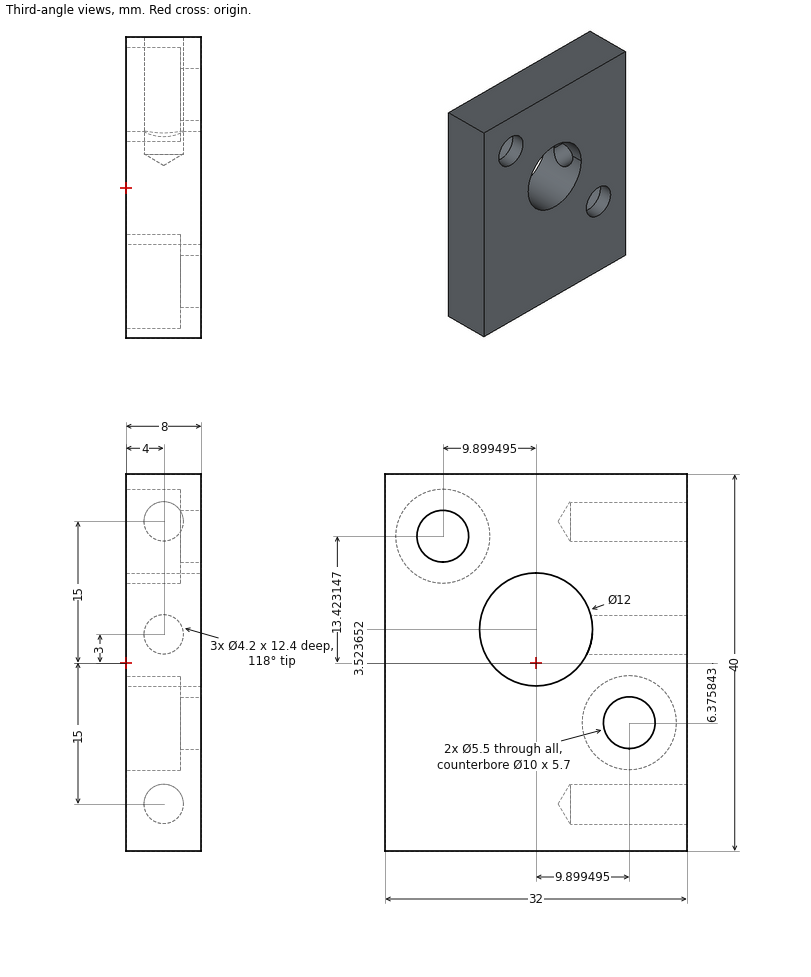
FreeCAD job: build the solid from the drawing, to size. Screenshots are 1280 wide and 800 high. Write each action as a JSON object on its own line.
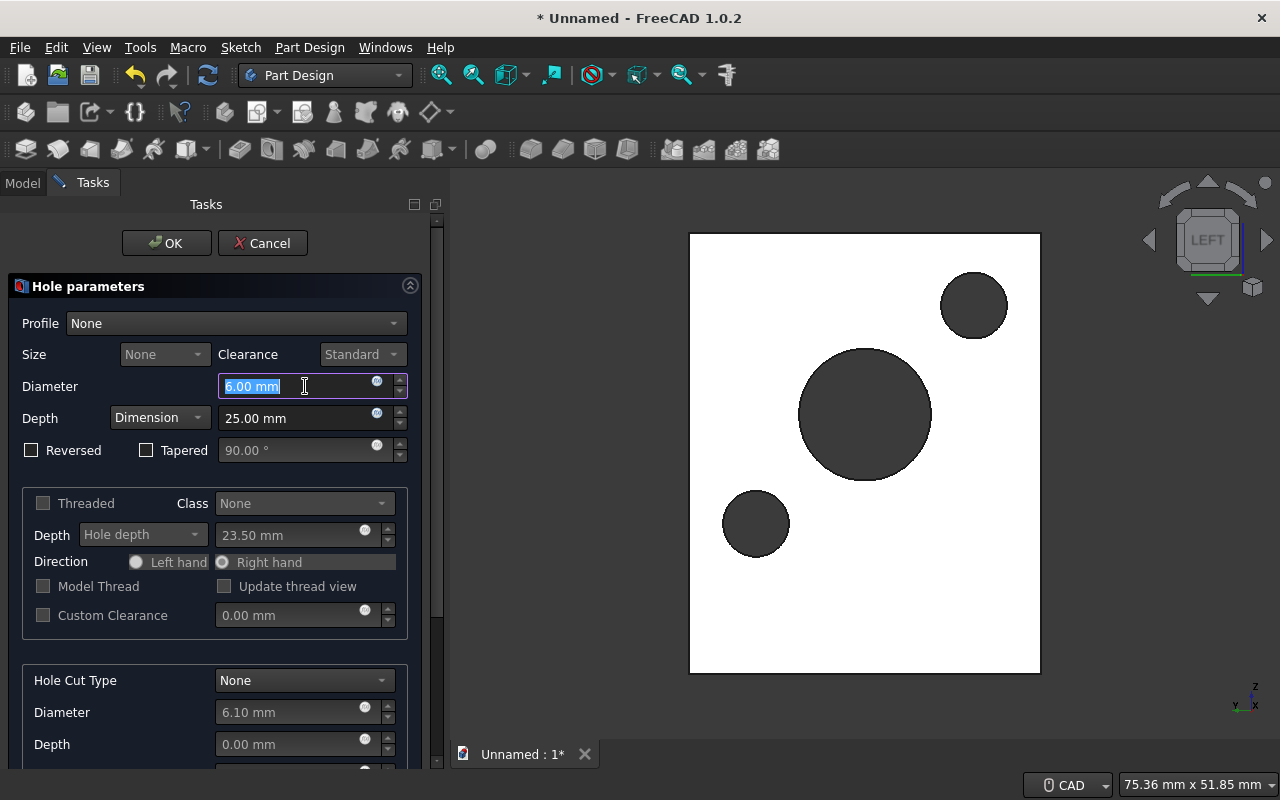
{"action": "type", "text": "5.5"}
{"action": "key", "text": "Tab"}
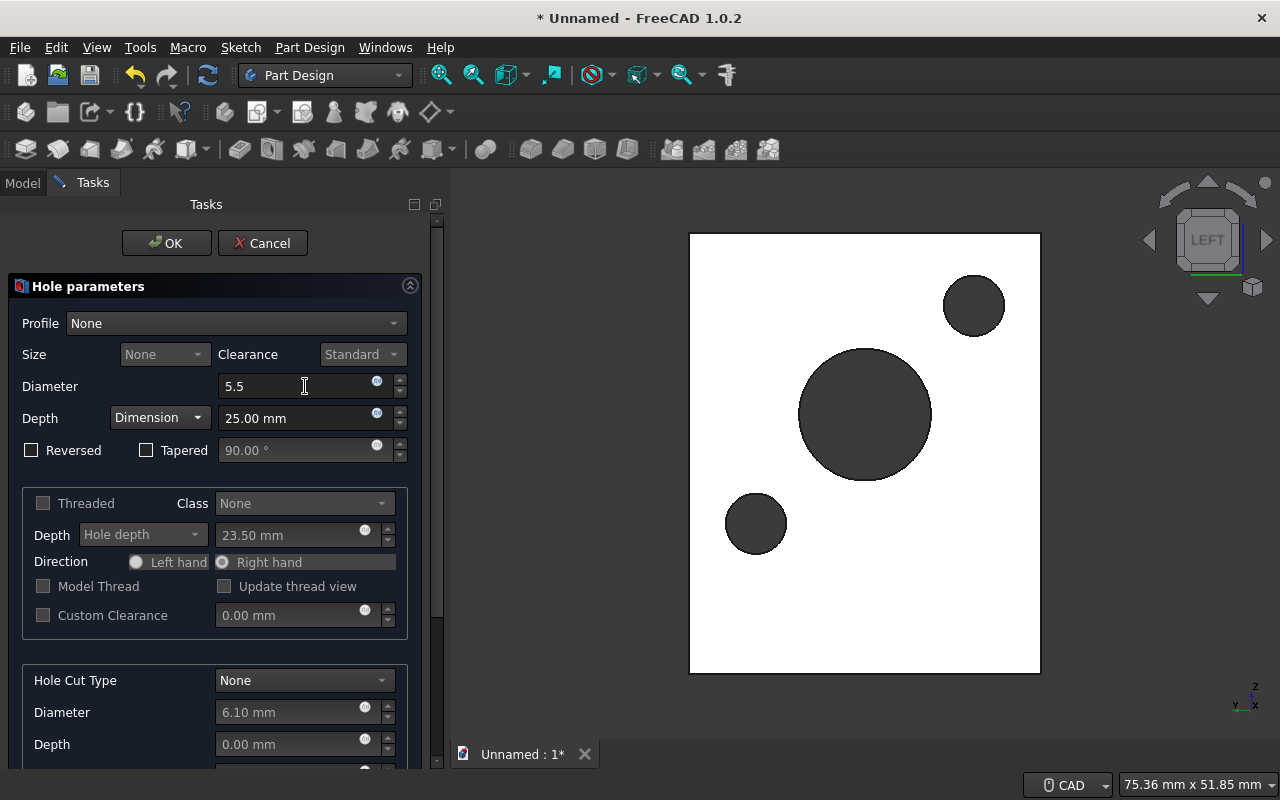
{"action": "left_click", "coordinate": [161, 418]}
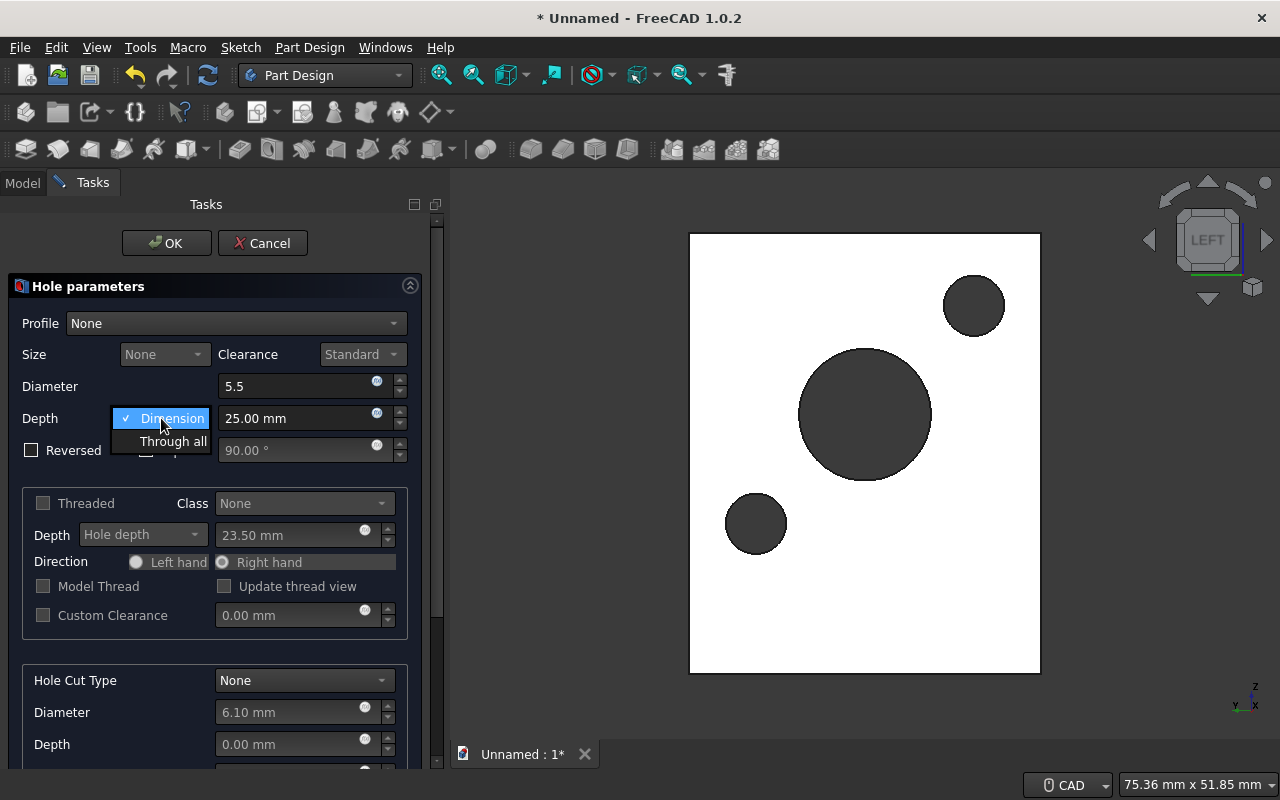
{"action": "left_click", "coordinate": [160, 442]}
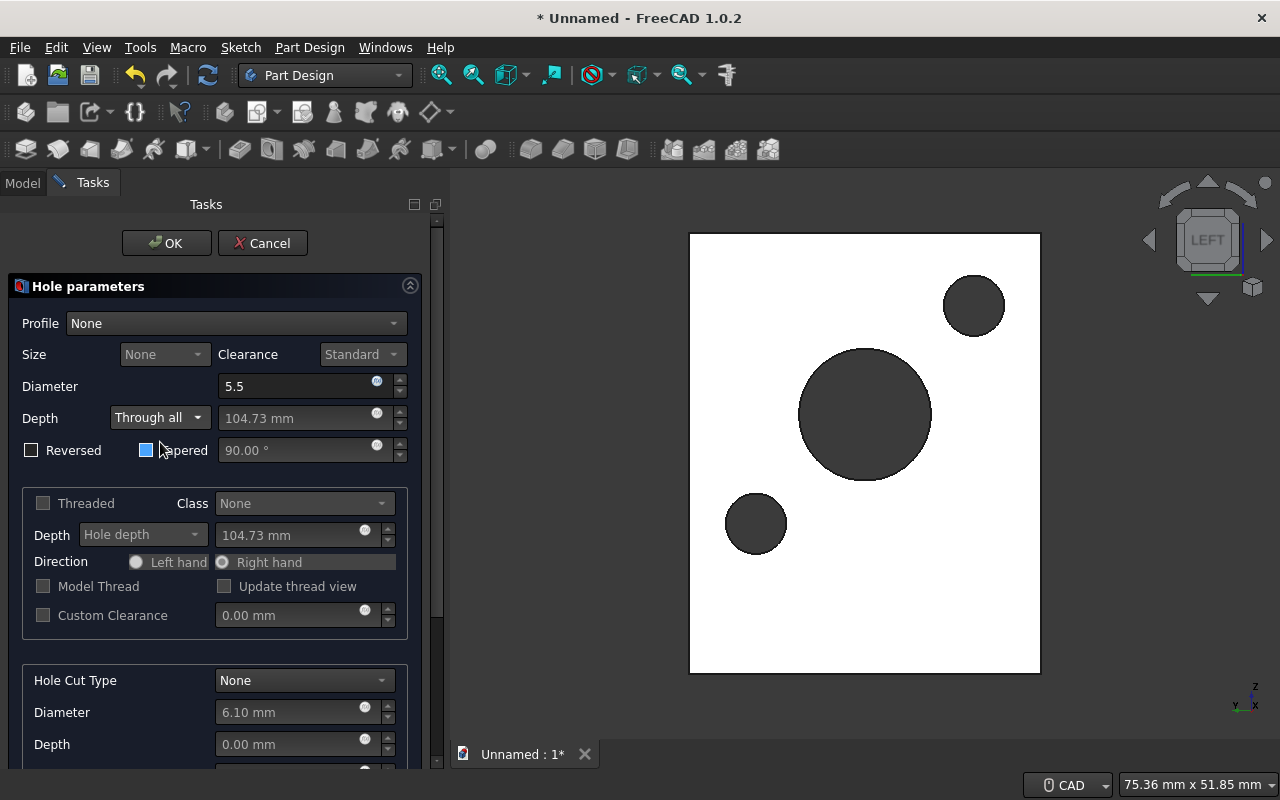
{"action": "left_click", "coordinate": [306, 680]}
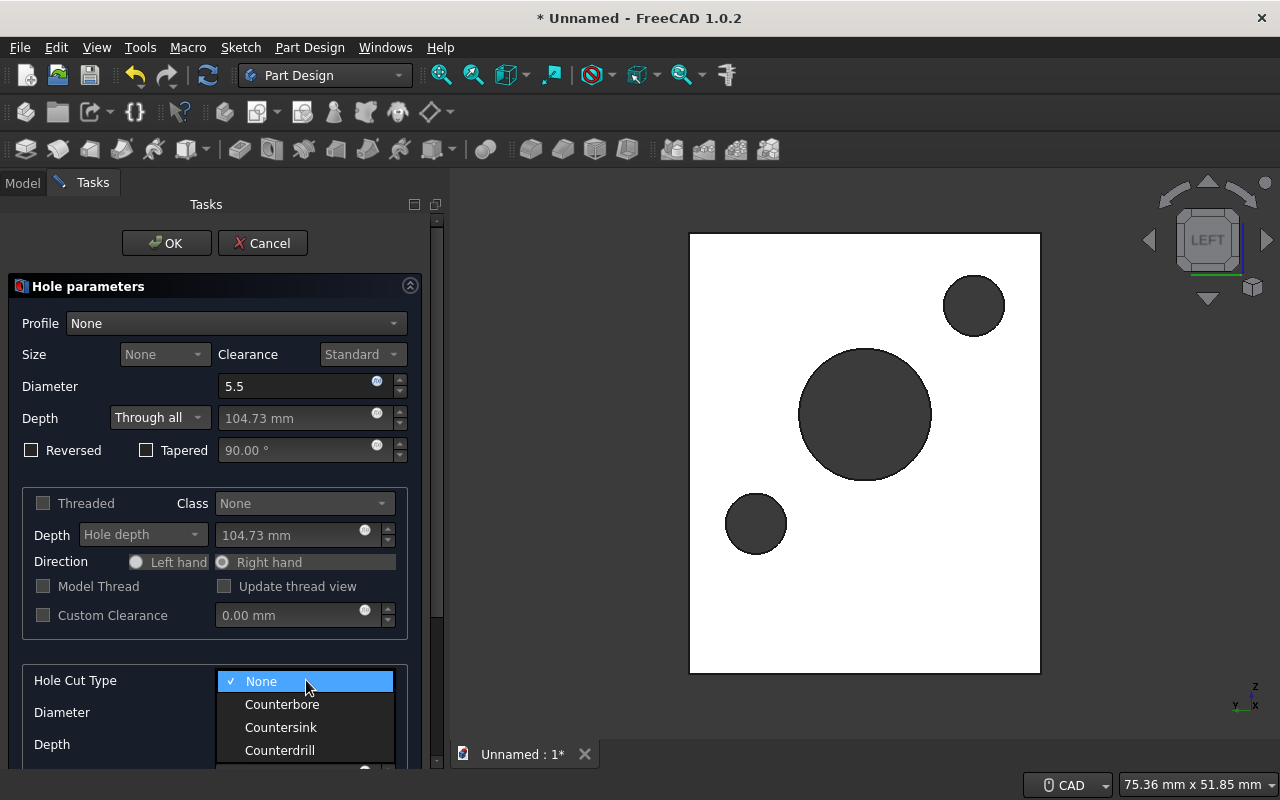
{"action": "left_click", "coordinate": [304, 704]}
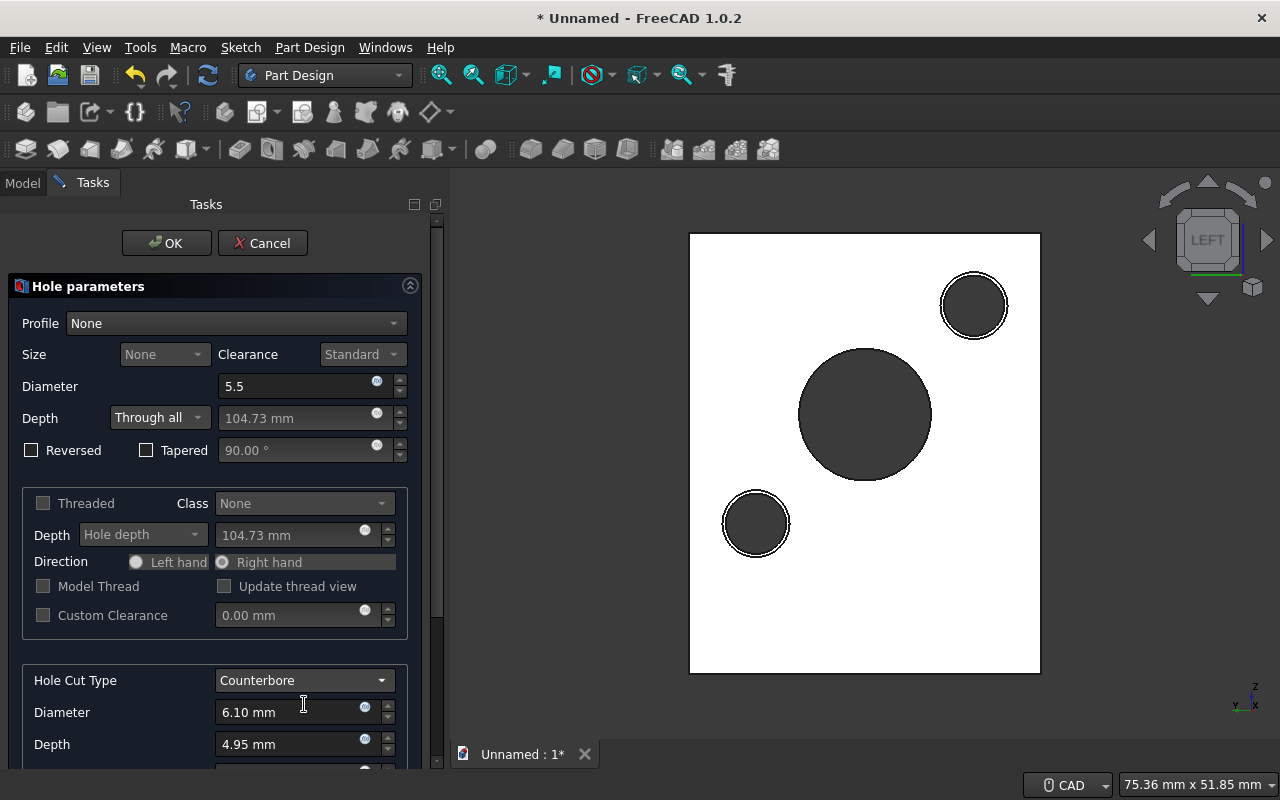
{"action": "triple_click", "coordinate": [298, 712]}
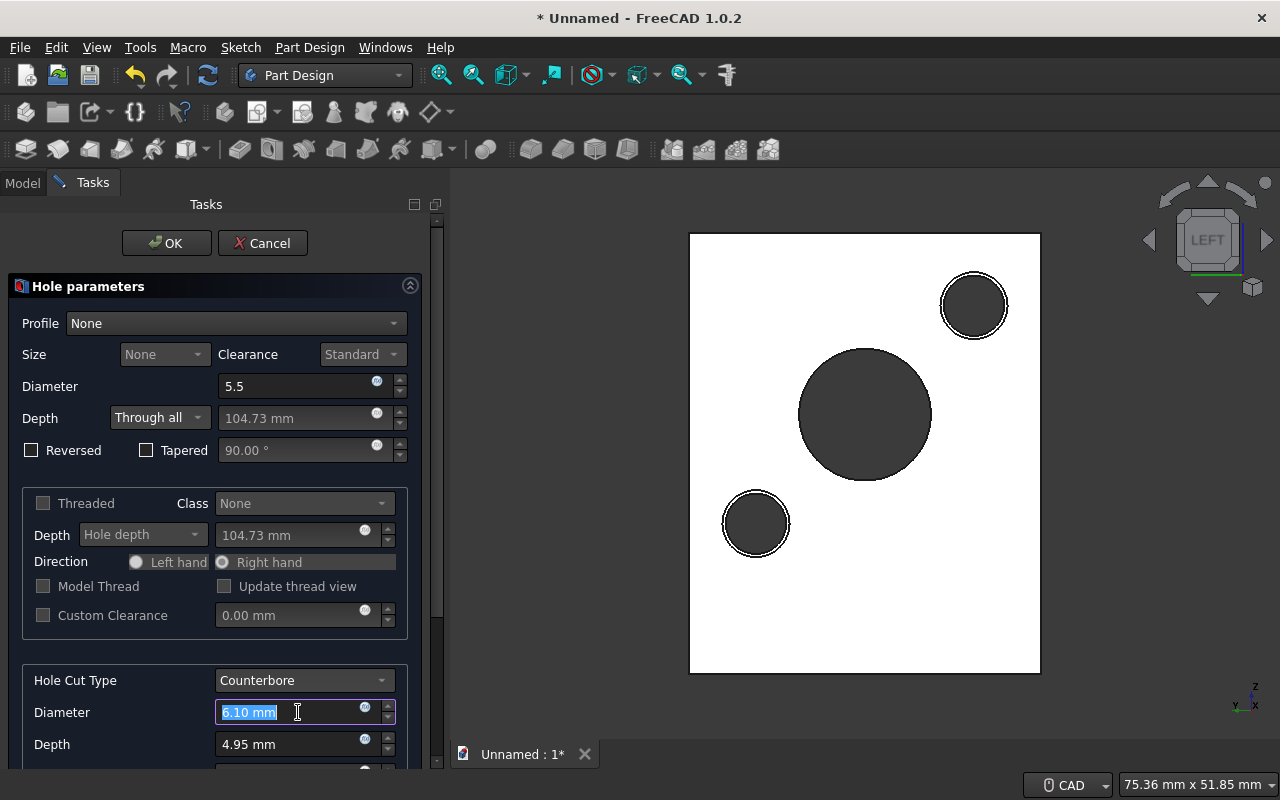
{"action": "type", "text": "10"}
{"action": "key", "text": "Tab"}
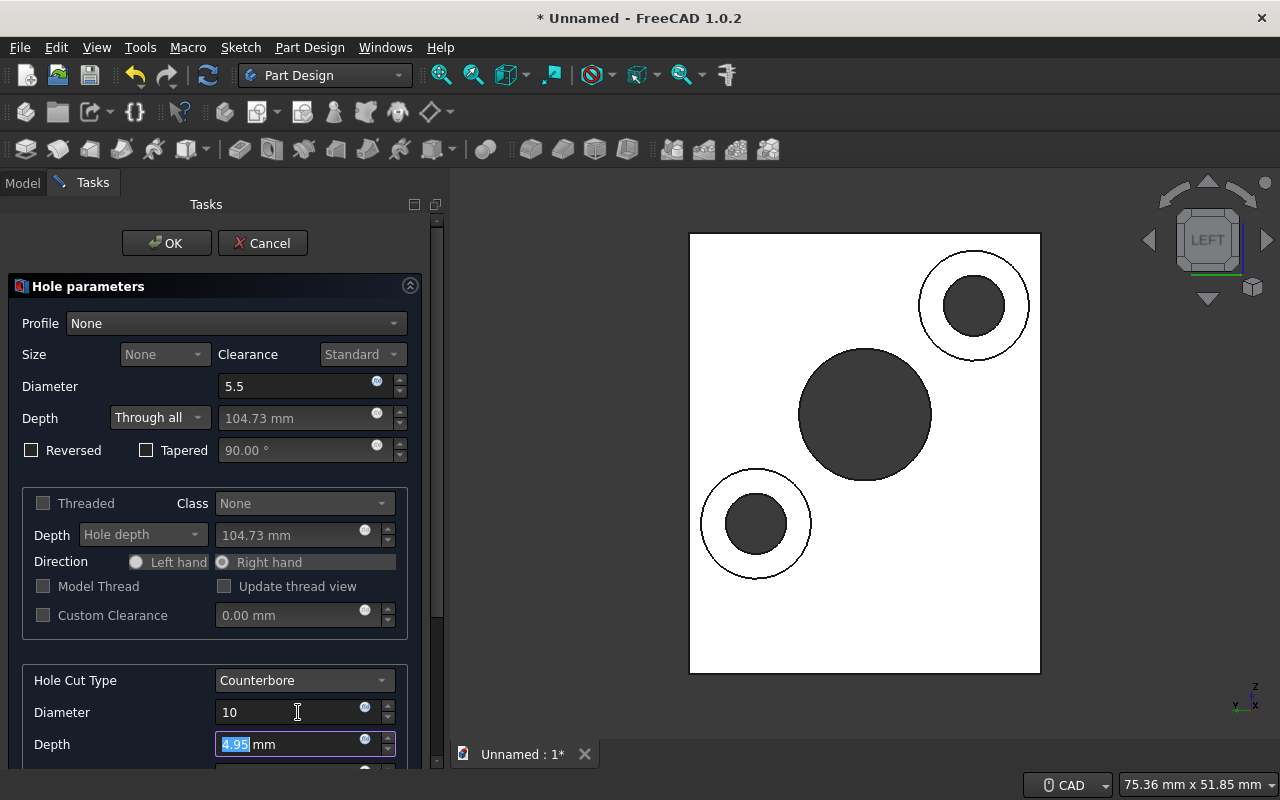
{"action": "type", "text": "5.7"}
{"action": "key", "text": "Tab"}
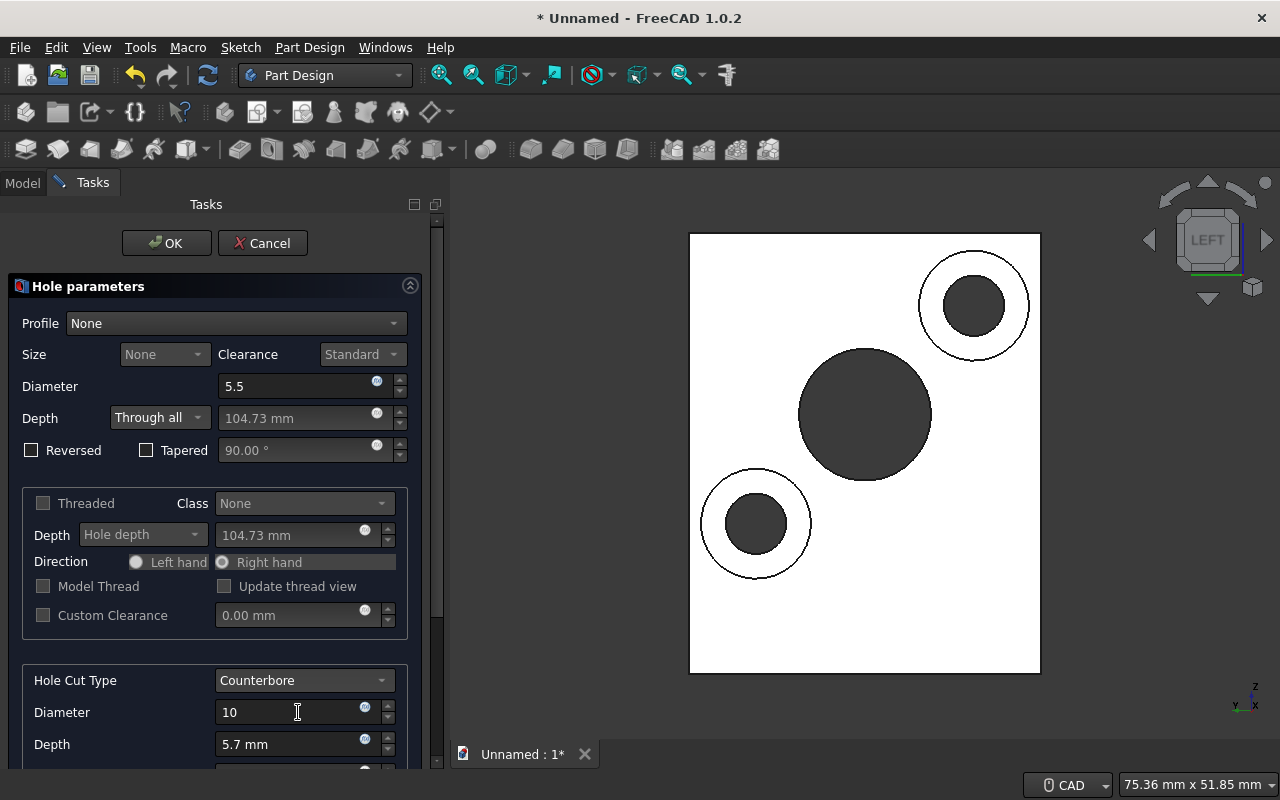
{"action": "left_click", "coordinate": [167, 243]}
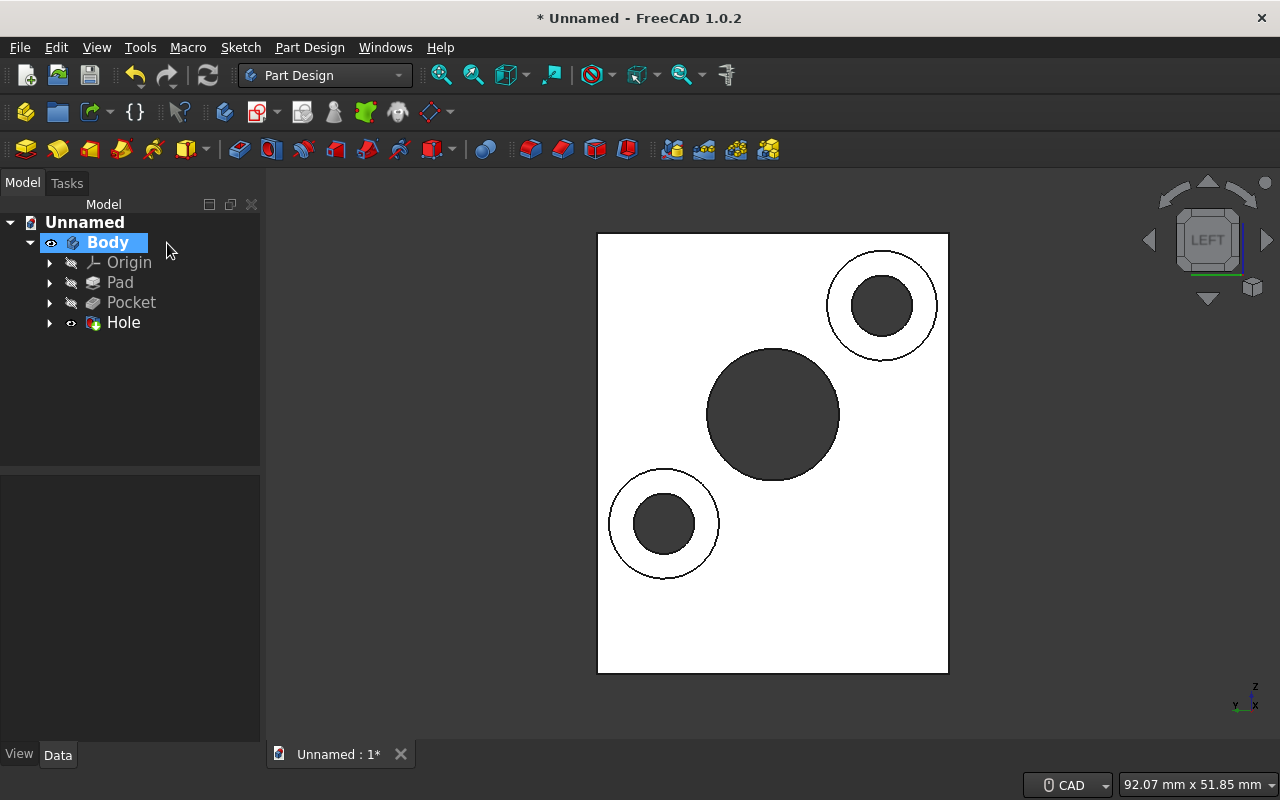
{"action": "key", "text": "4"}